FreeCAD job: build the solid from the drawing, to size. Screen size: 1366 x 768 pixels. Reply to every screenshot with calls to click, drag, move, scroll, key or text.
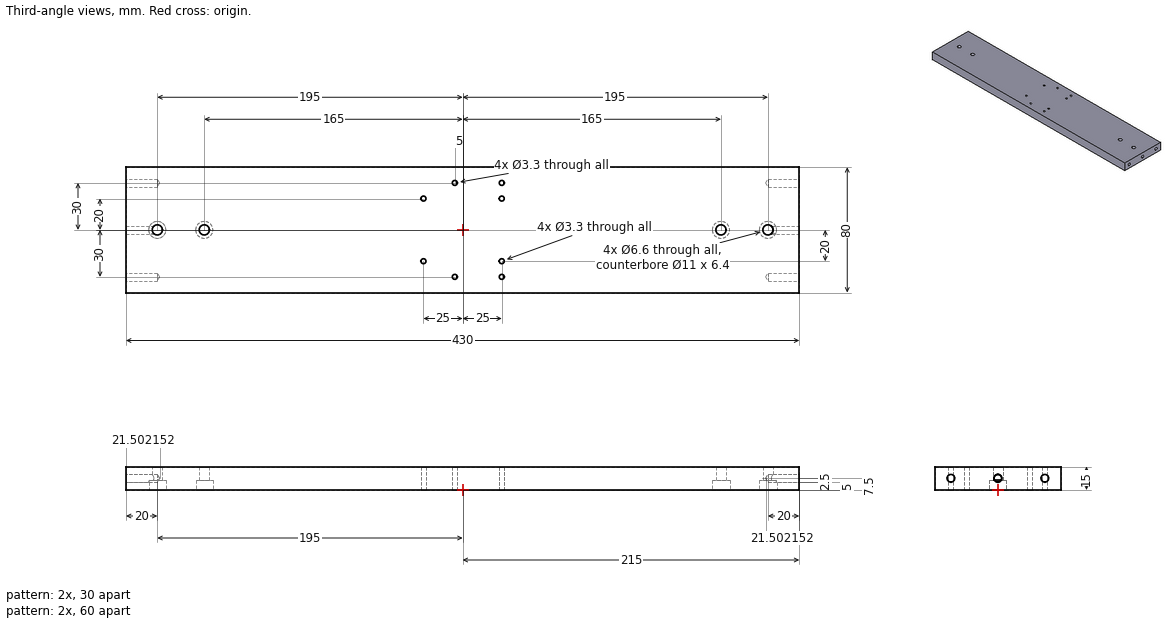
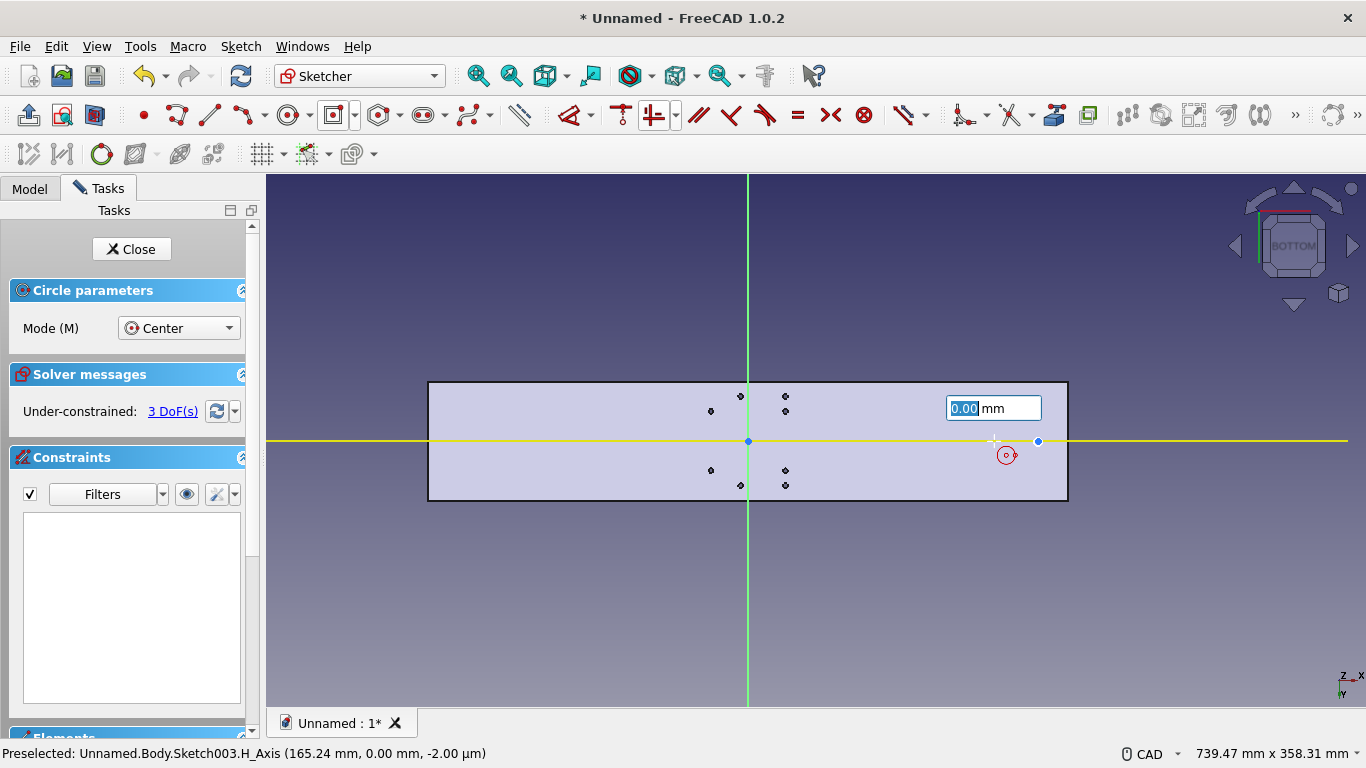
scroll(992, 446, up, 7)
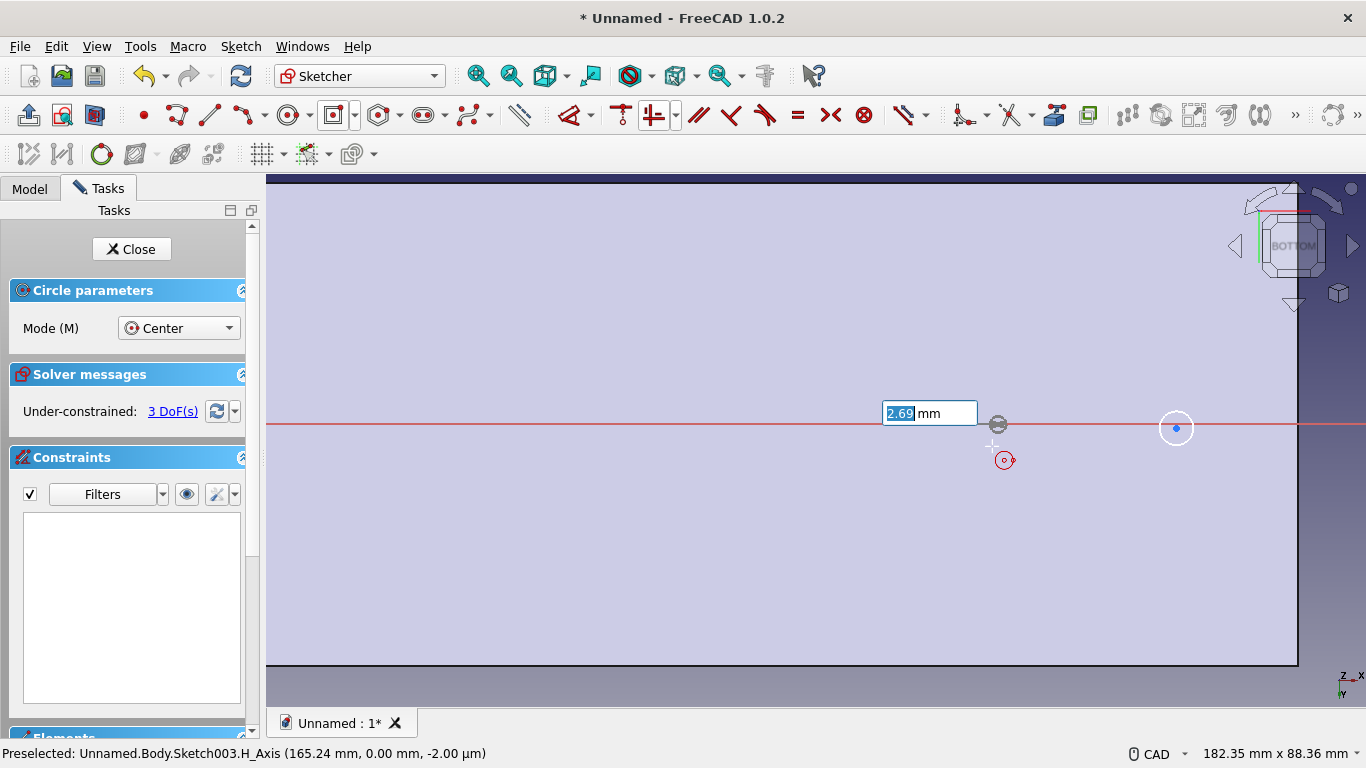
click(990, 443)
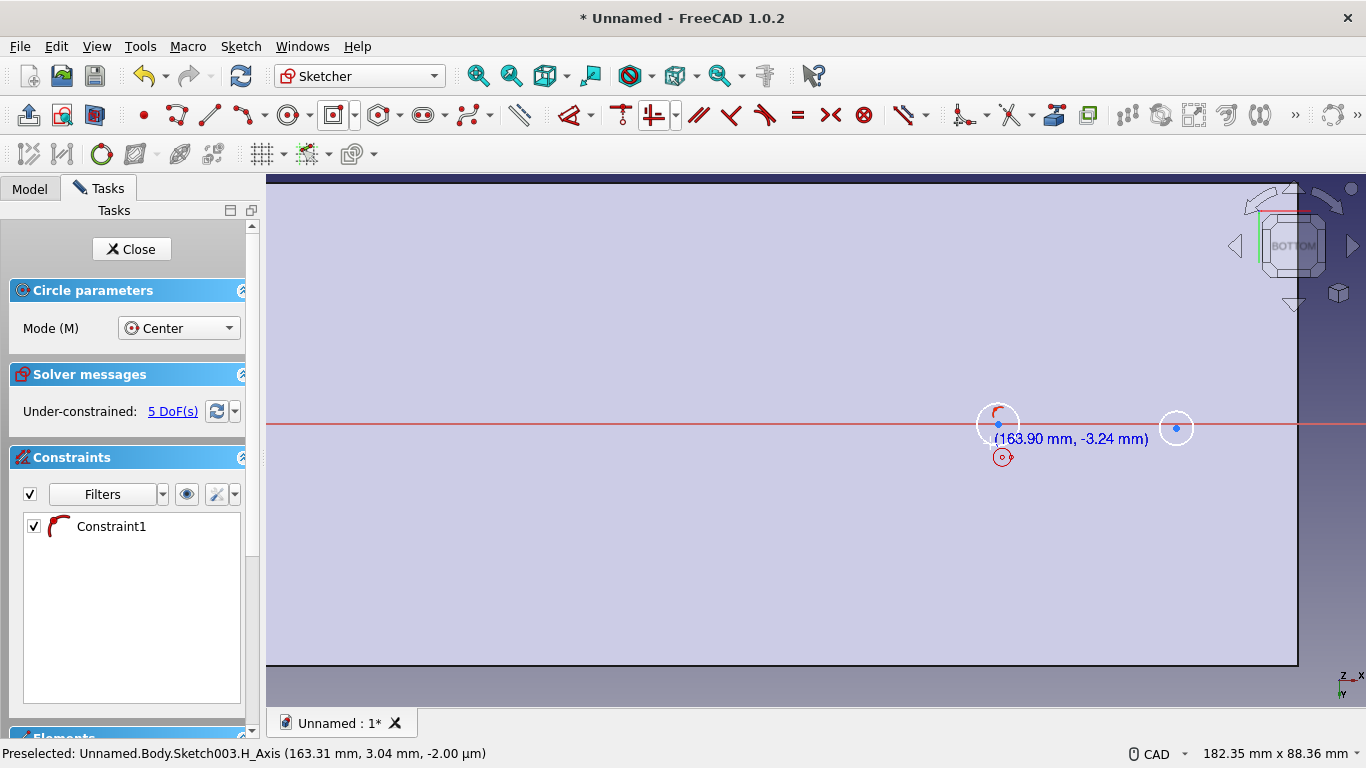
scroll(992, 446, down, 7)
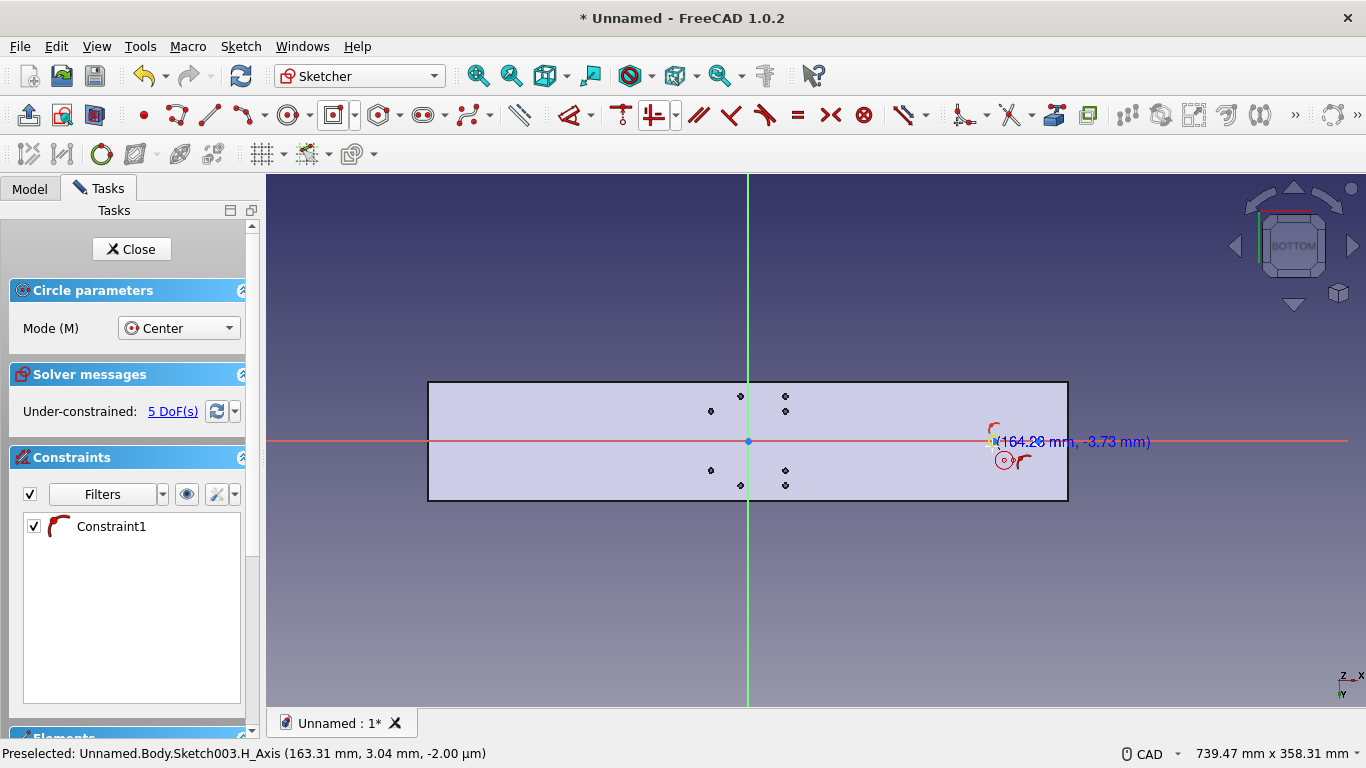
scroll(503, 441, up, 8)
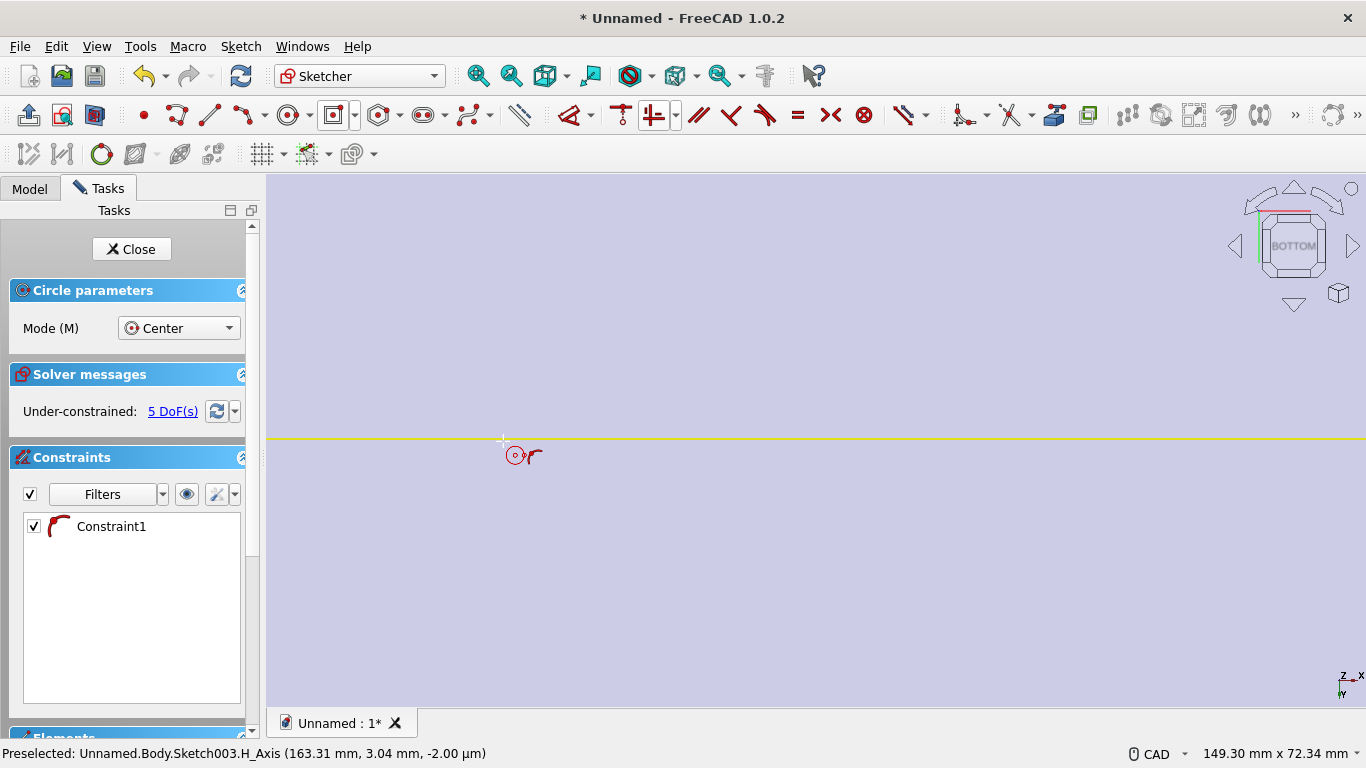
scroll(502, 441, down, 8)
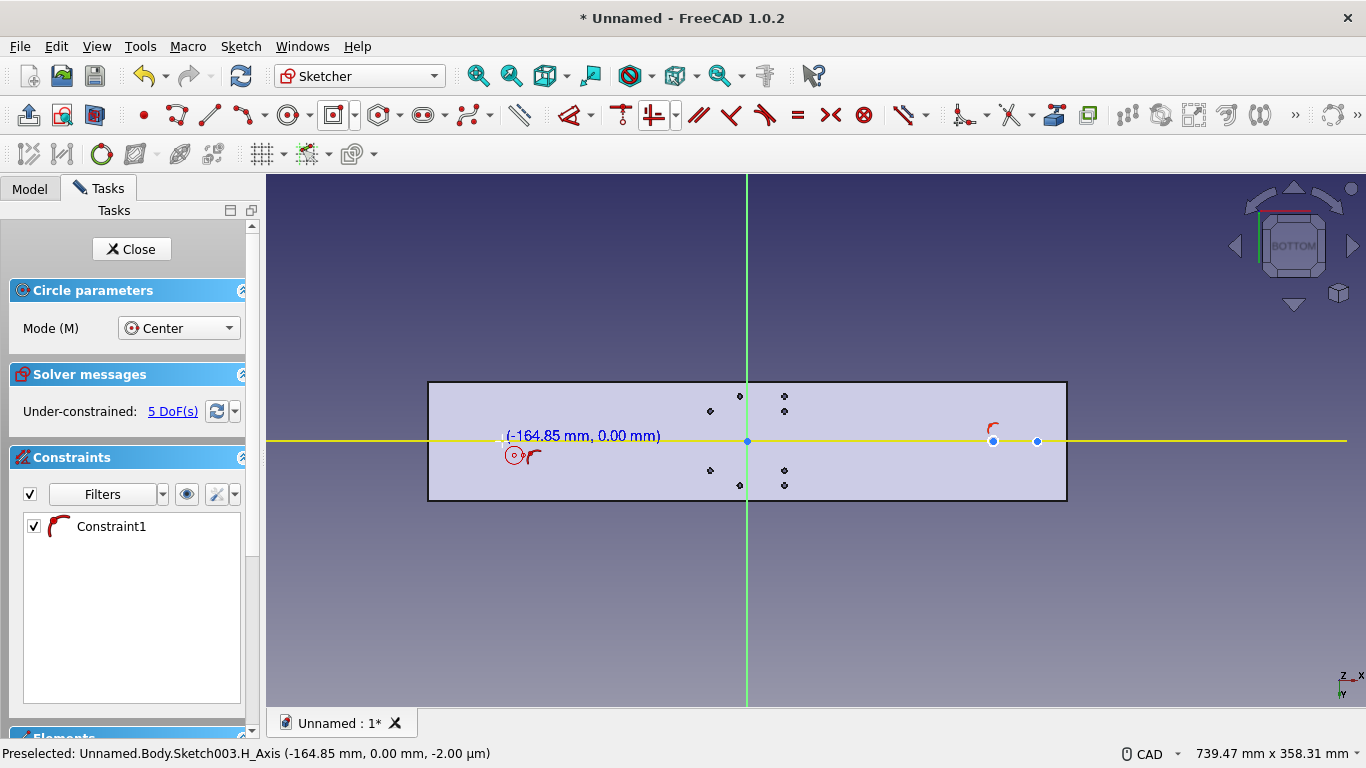
click(502, 441)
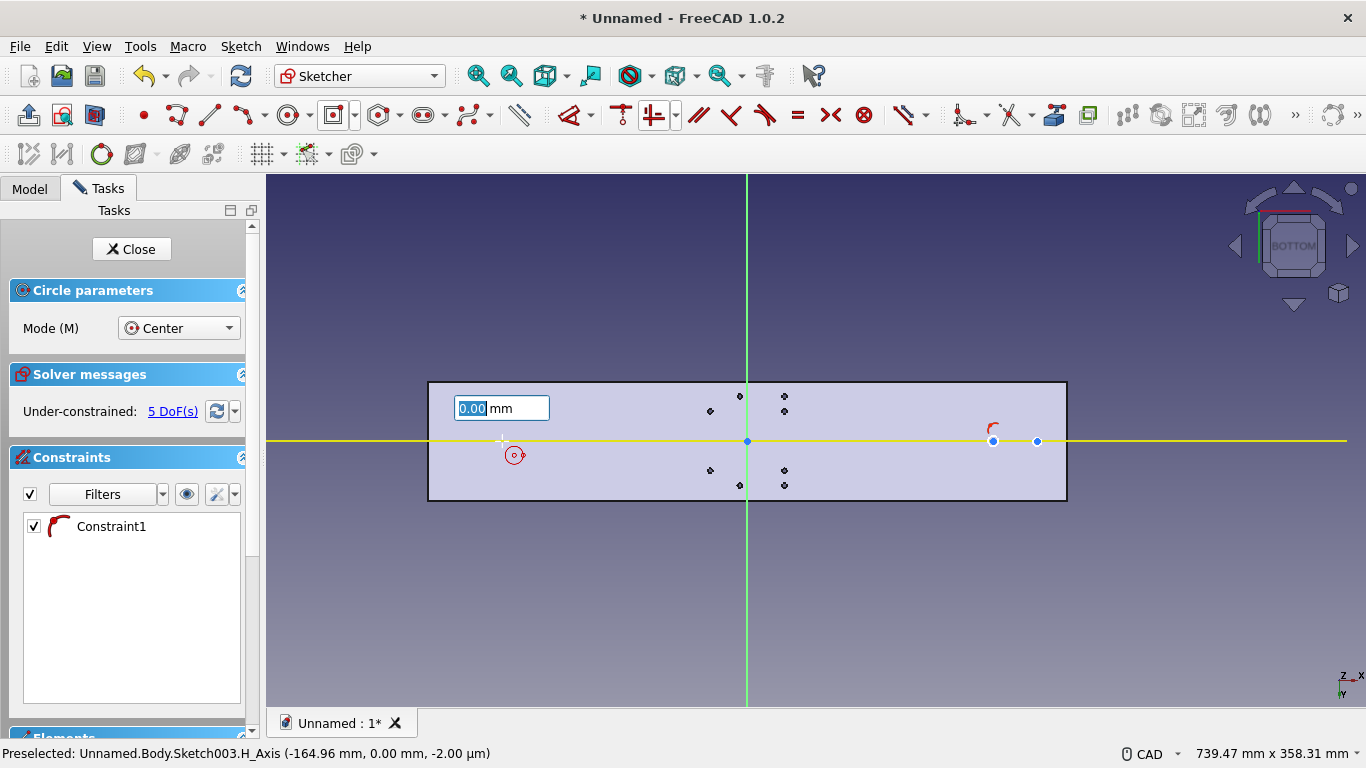
scroll(504, 436, up, 7)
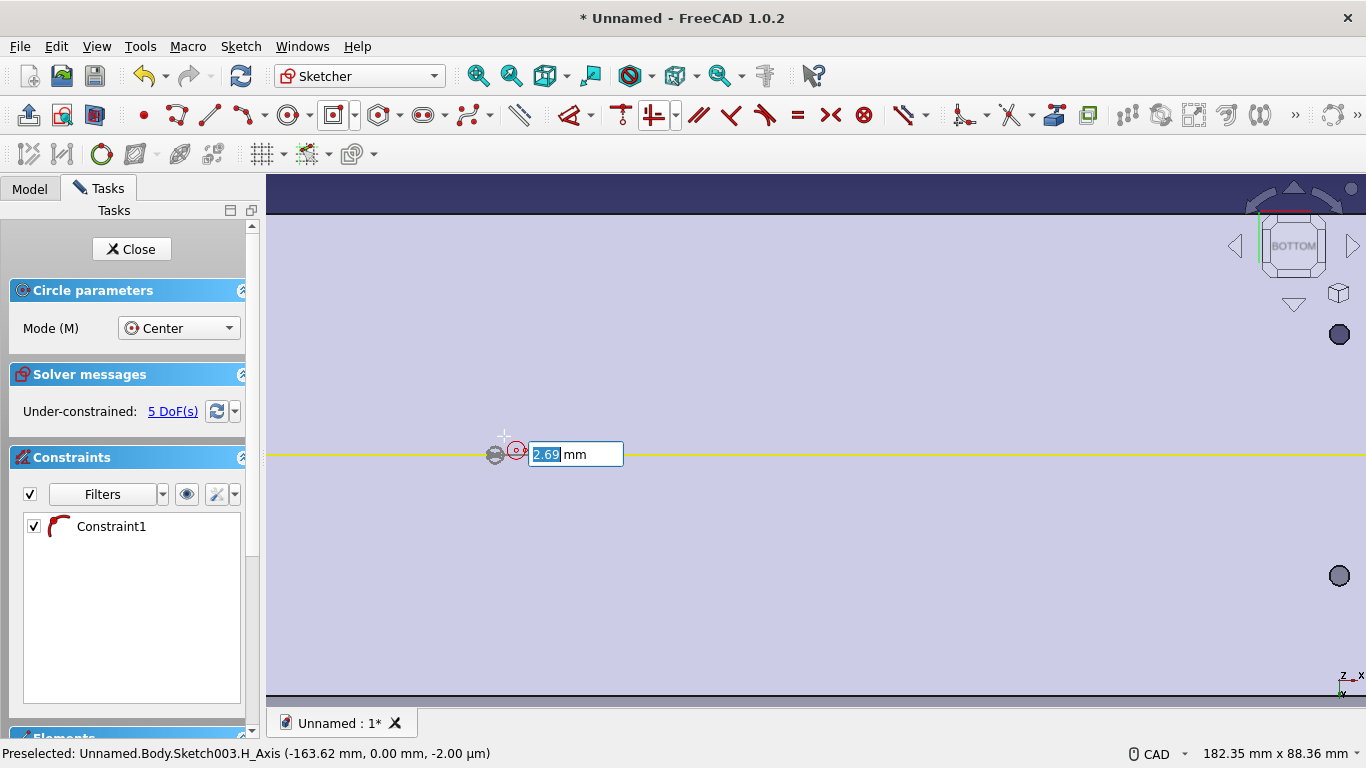
click(502, 436)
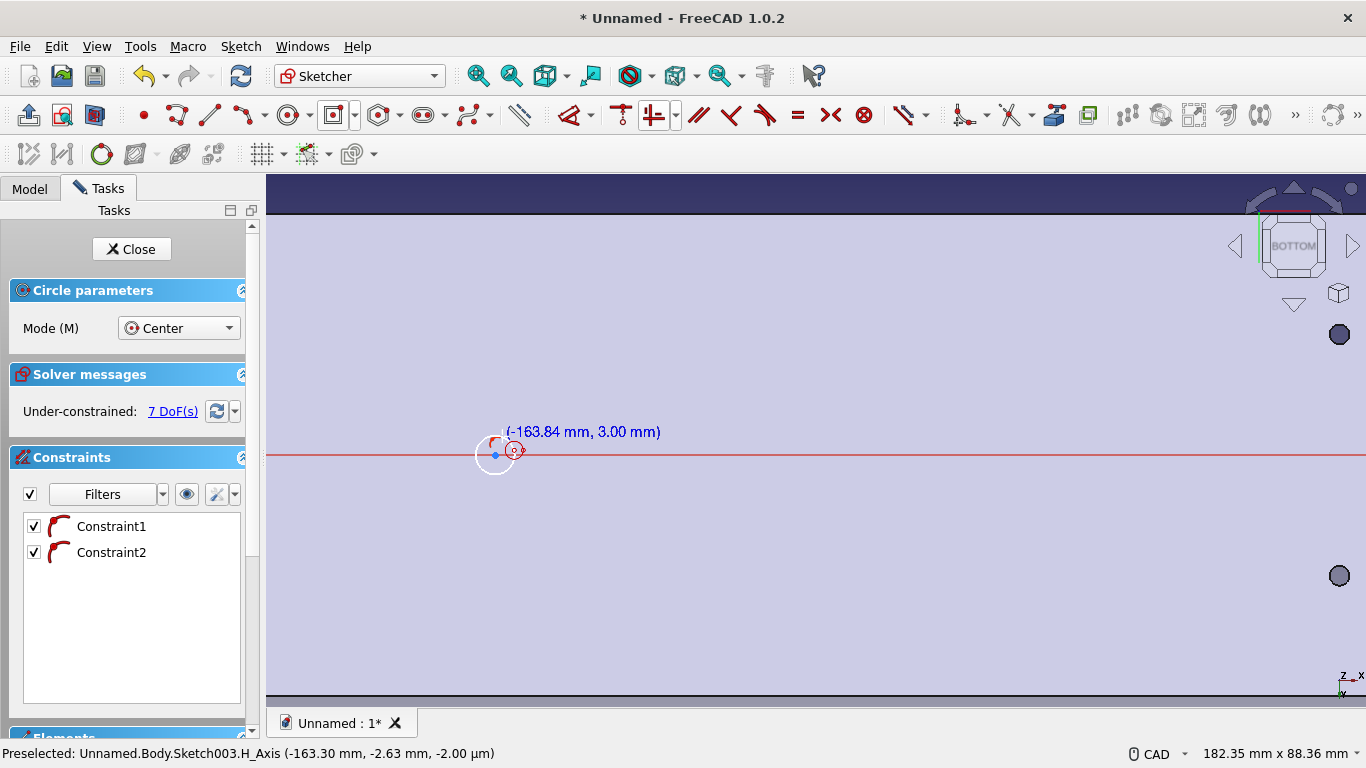
scroll(504, 436, down, 7)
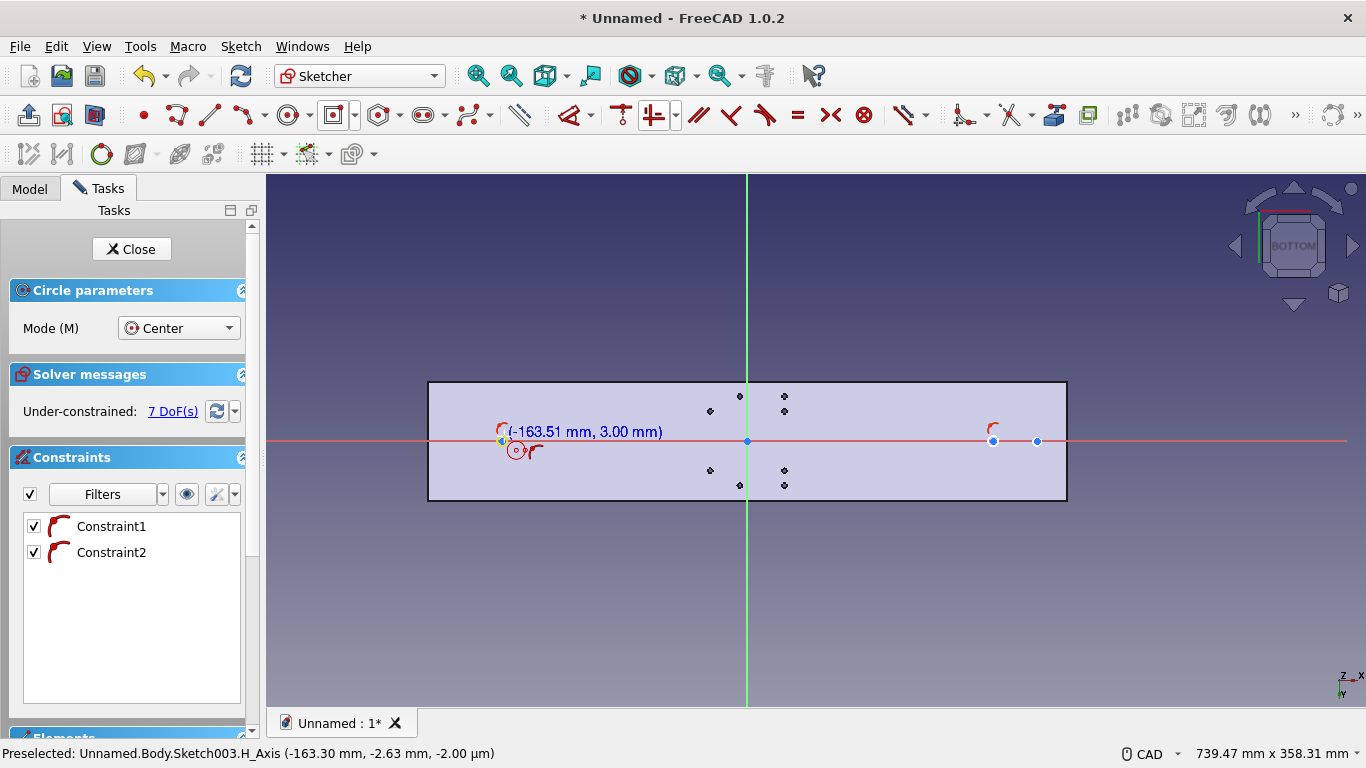
click(457, 441)